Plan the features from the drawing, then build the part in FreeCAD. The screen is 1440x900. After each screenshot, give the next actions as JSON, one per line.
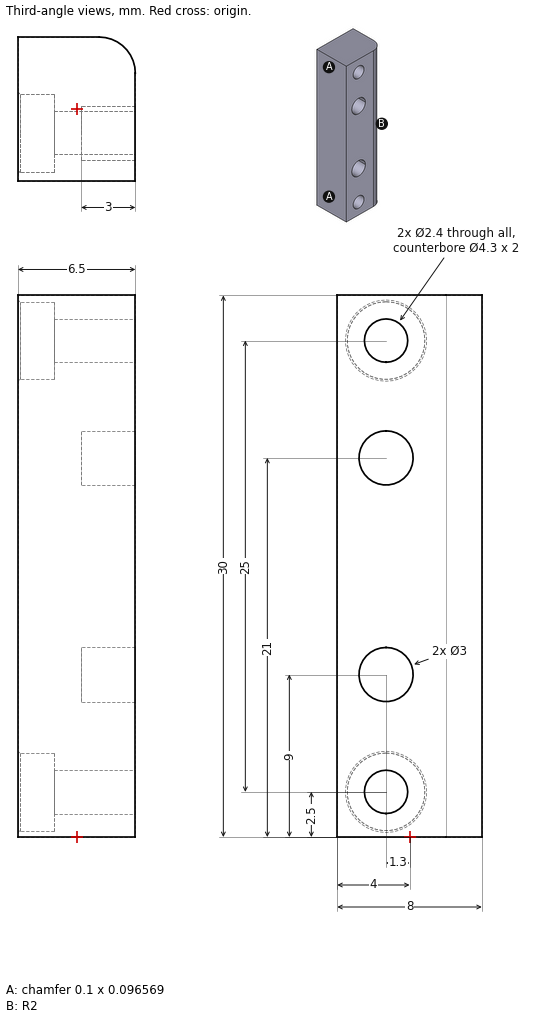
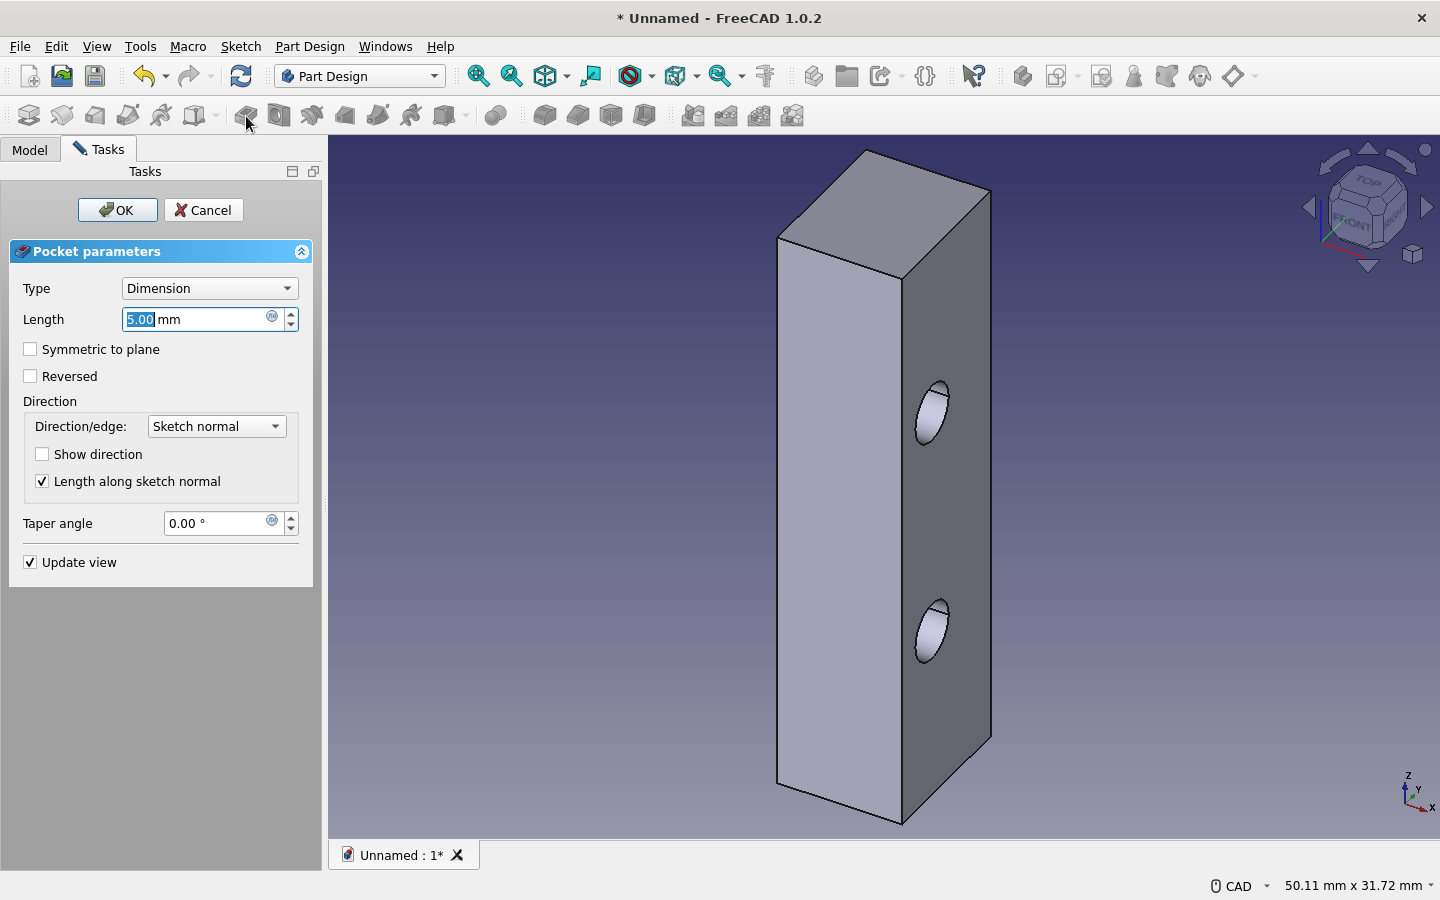
{"action": "type", "text": "3"}
{"action": "key", "text": "Tab"}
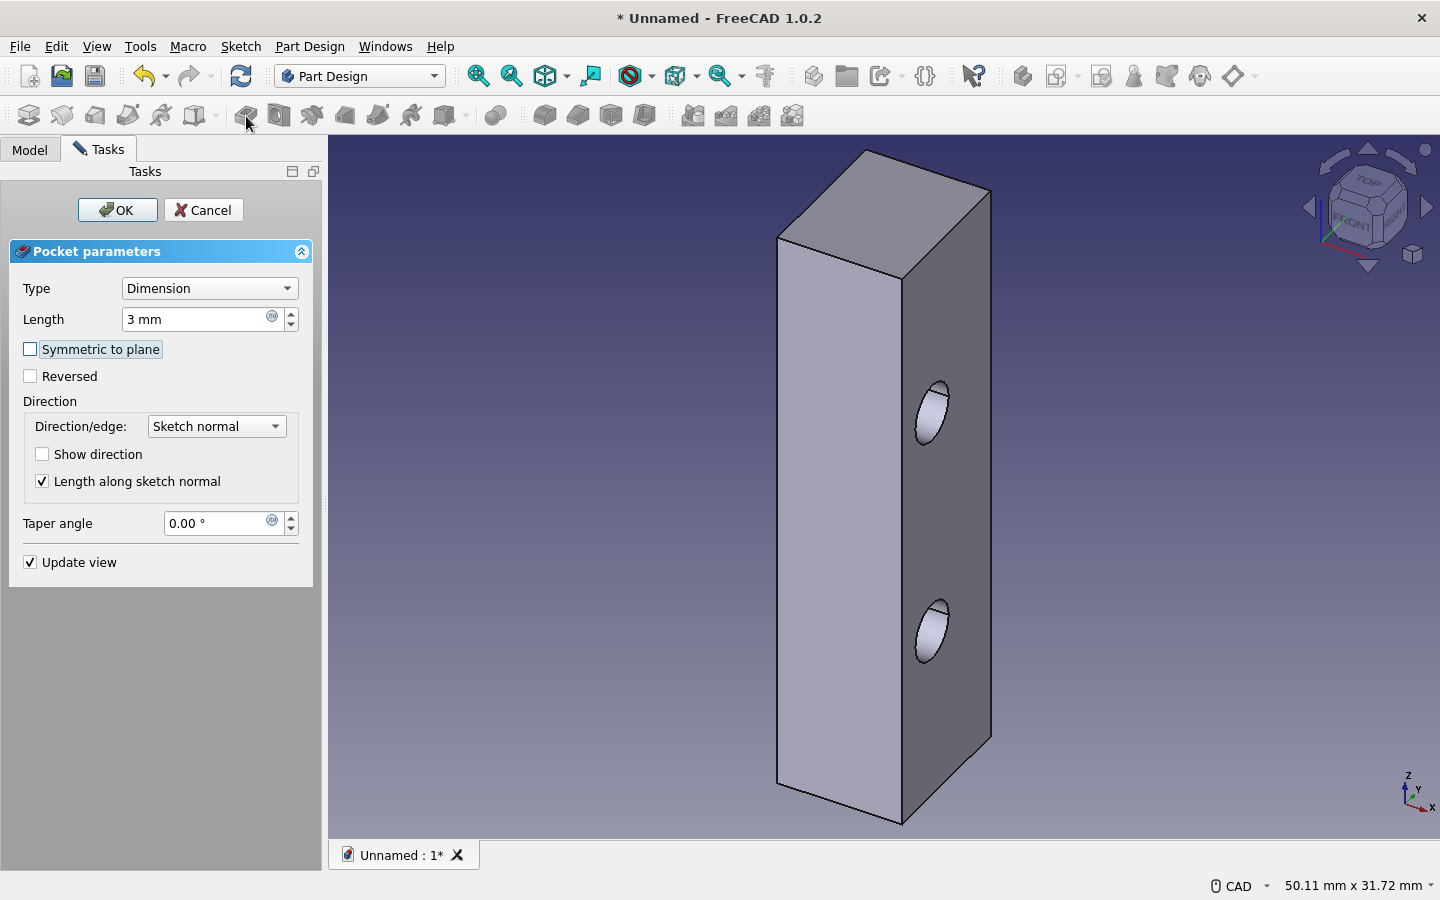
{"action": "left_click", "coordinate": [118, 210]}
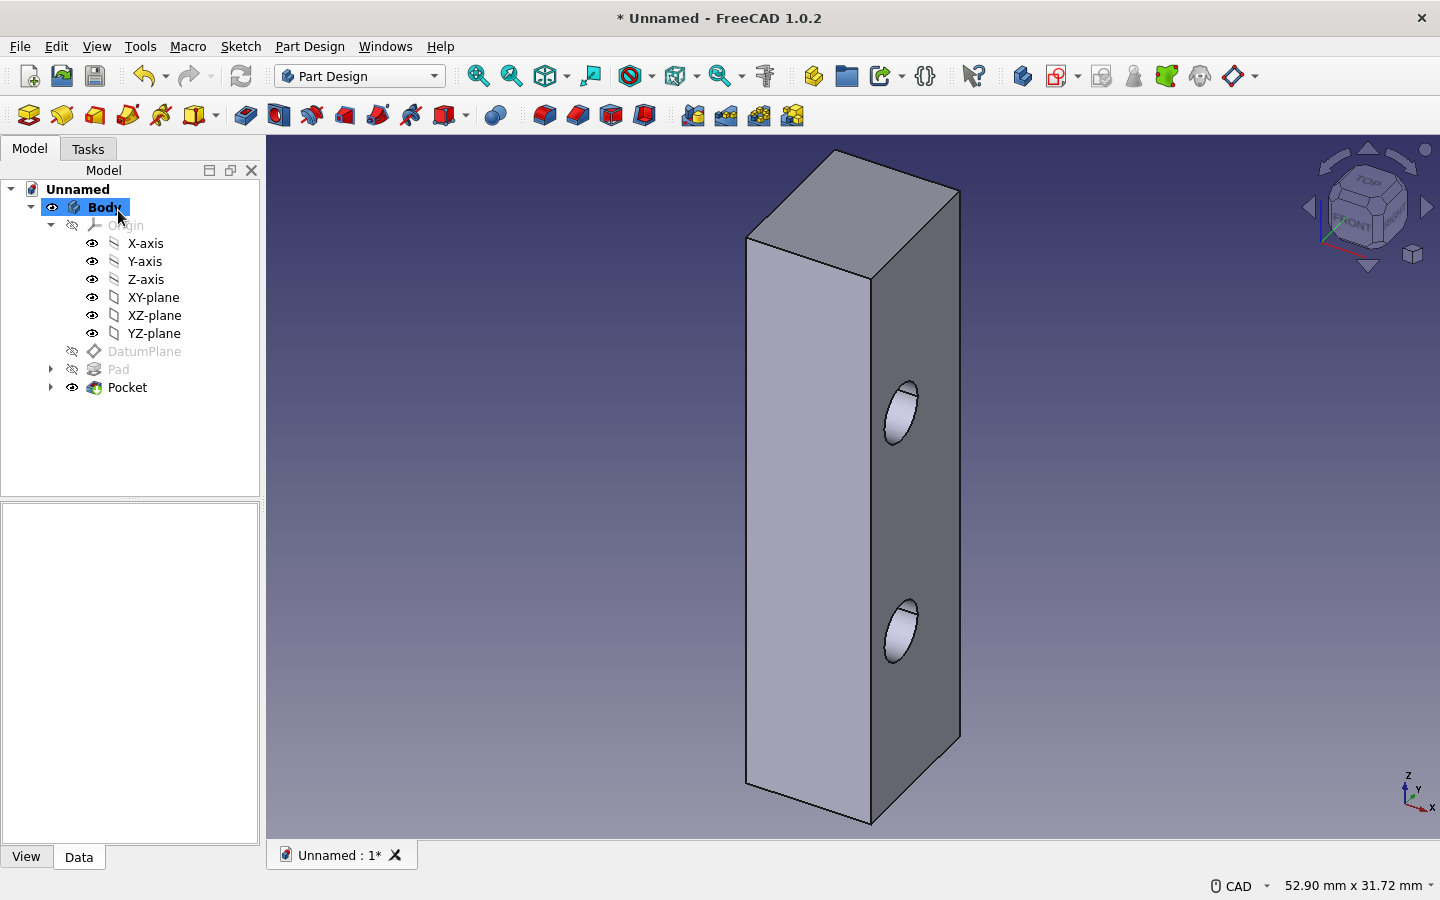
{"action": "key", "text": "6"}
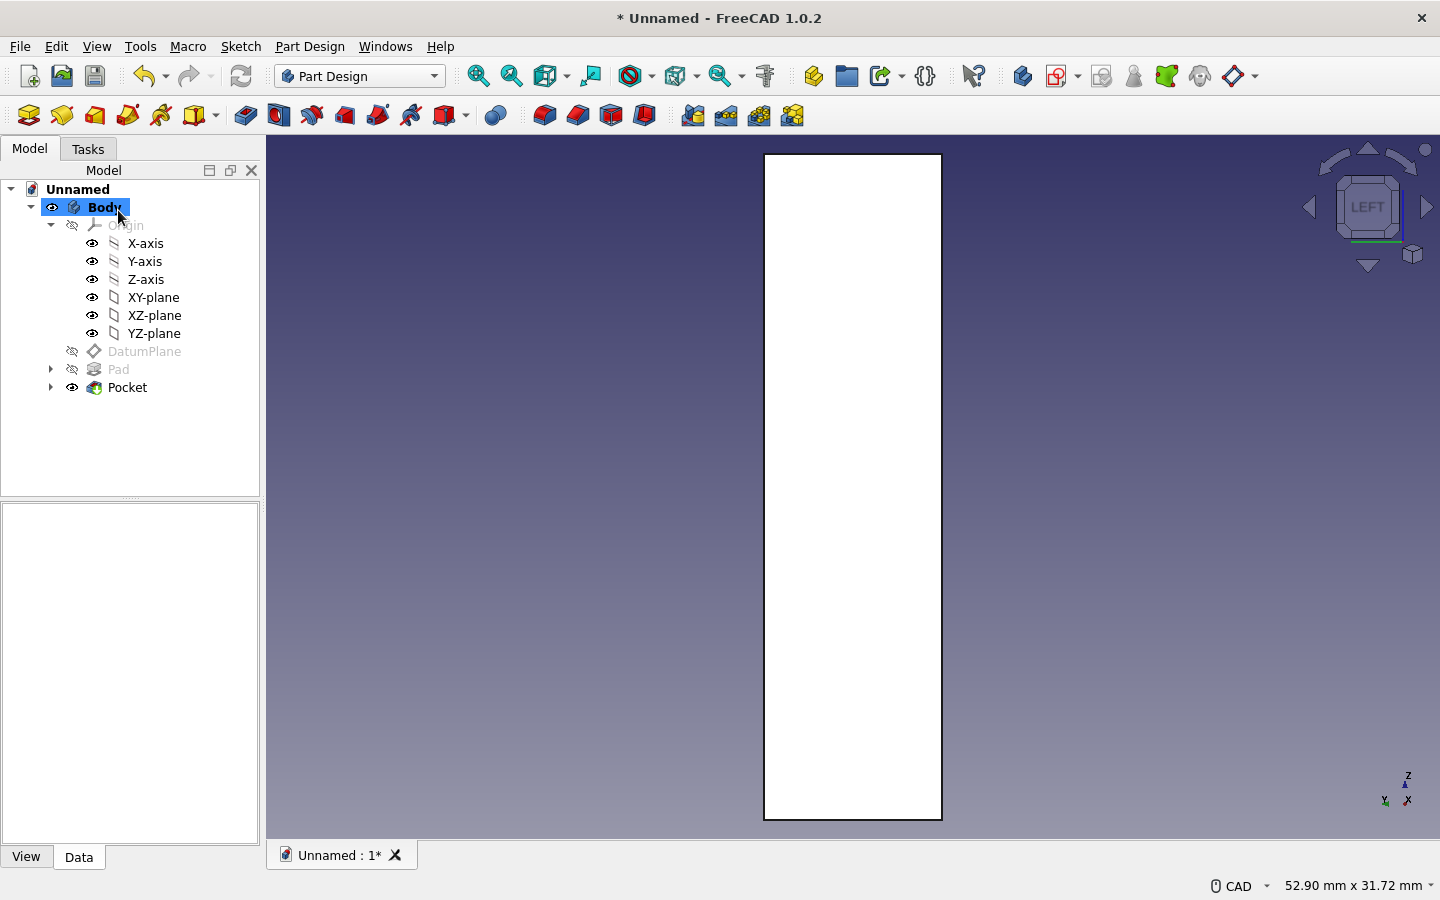
{"action": "left_click", "coordinate": [853, 296]}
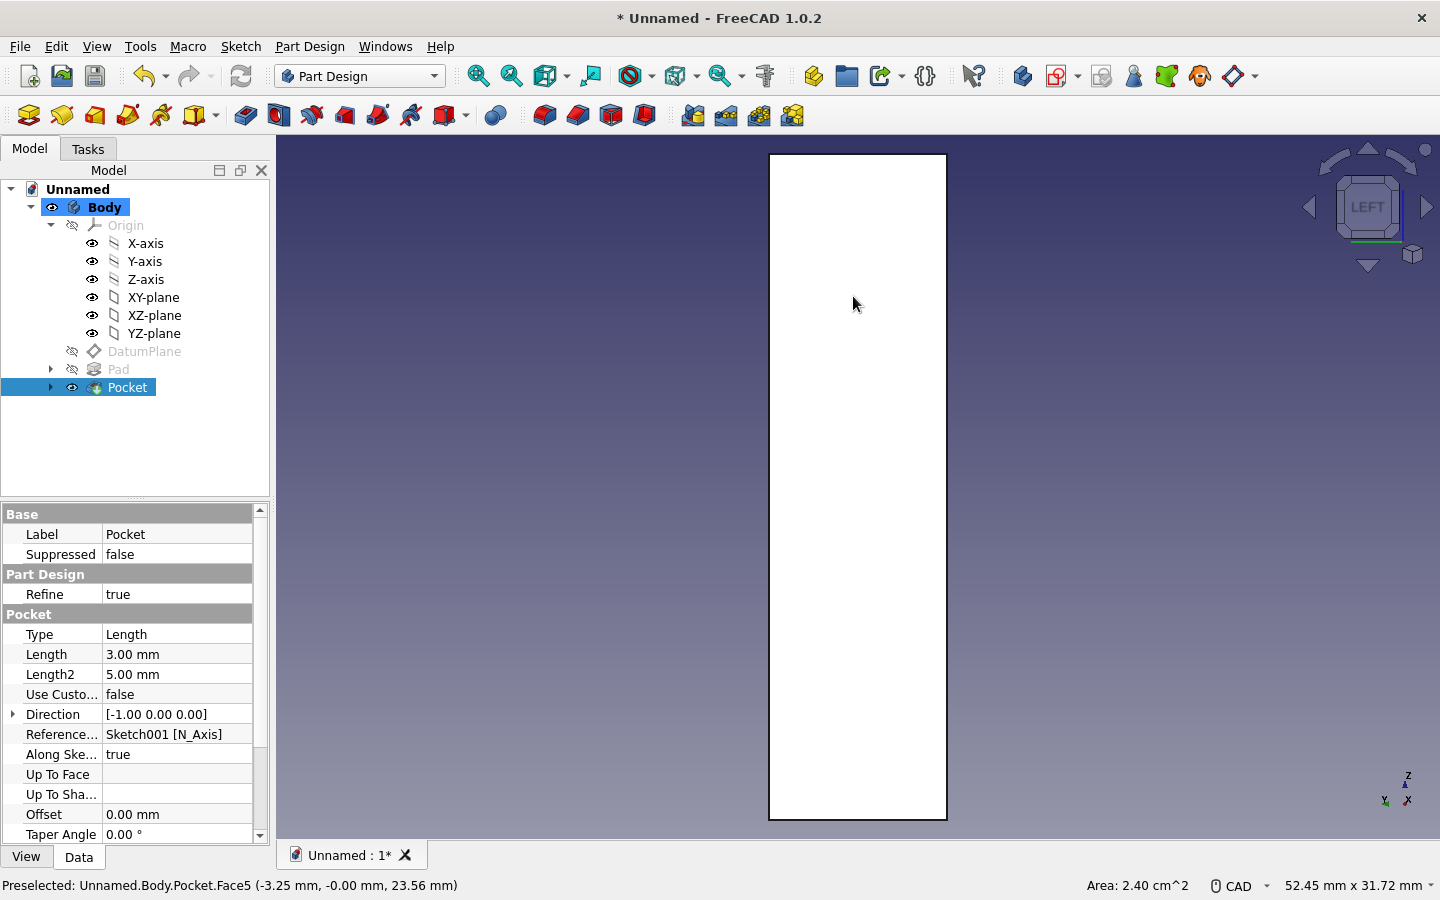
{"action": "left_click", "coordinate": [1056, 76]}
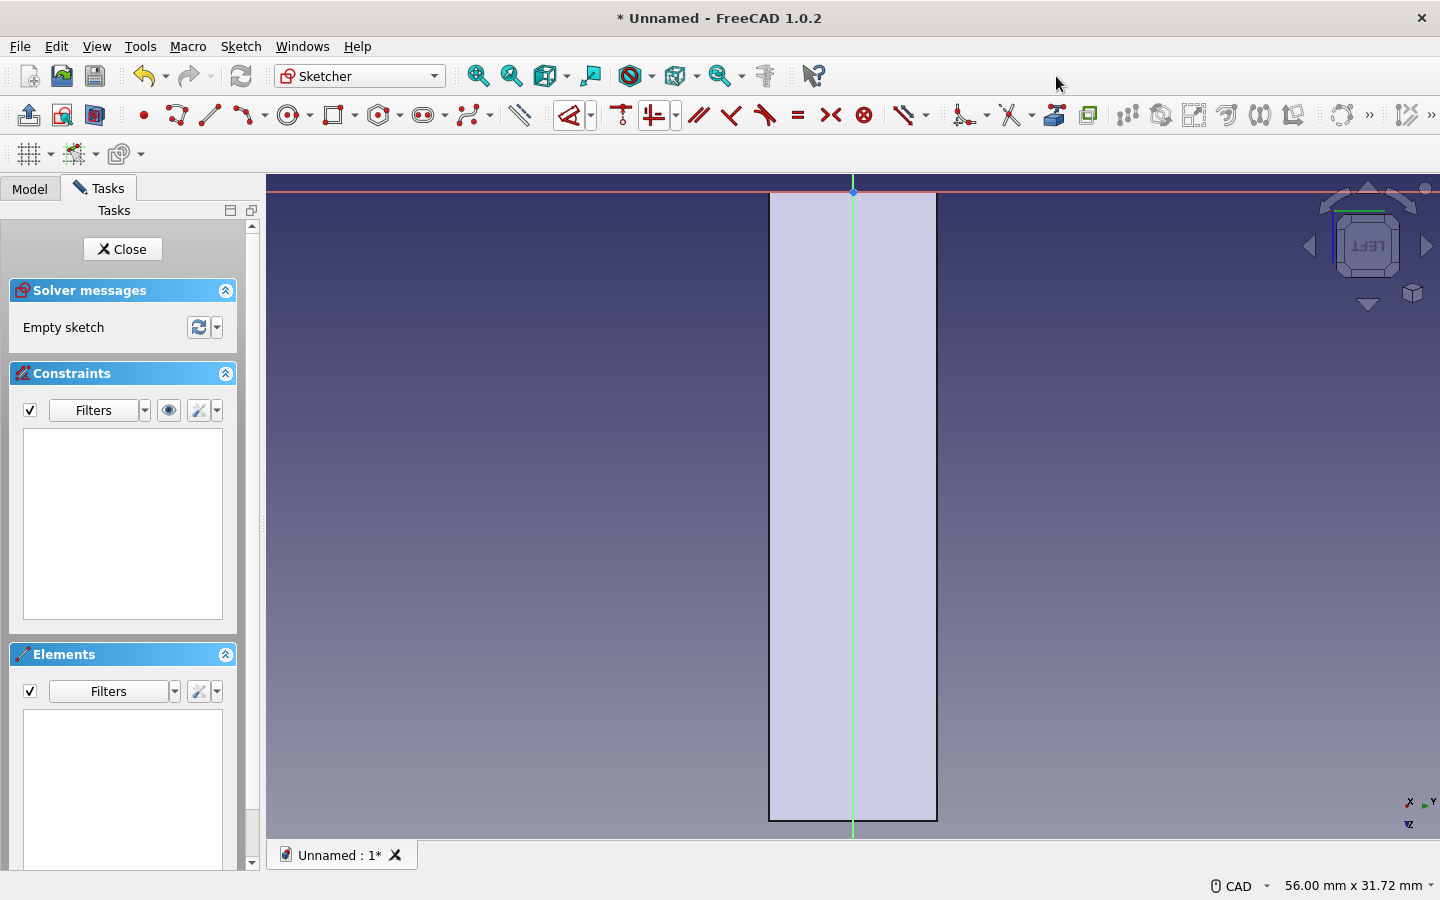
{"action": "scroll", "coordinate": [699, 534], "scroll_direction": "down", "scroll_amount": 2}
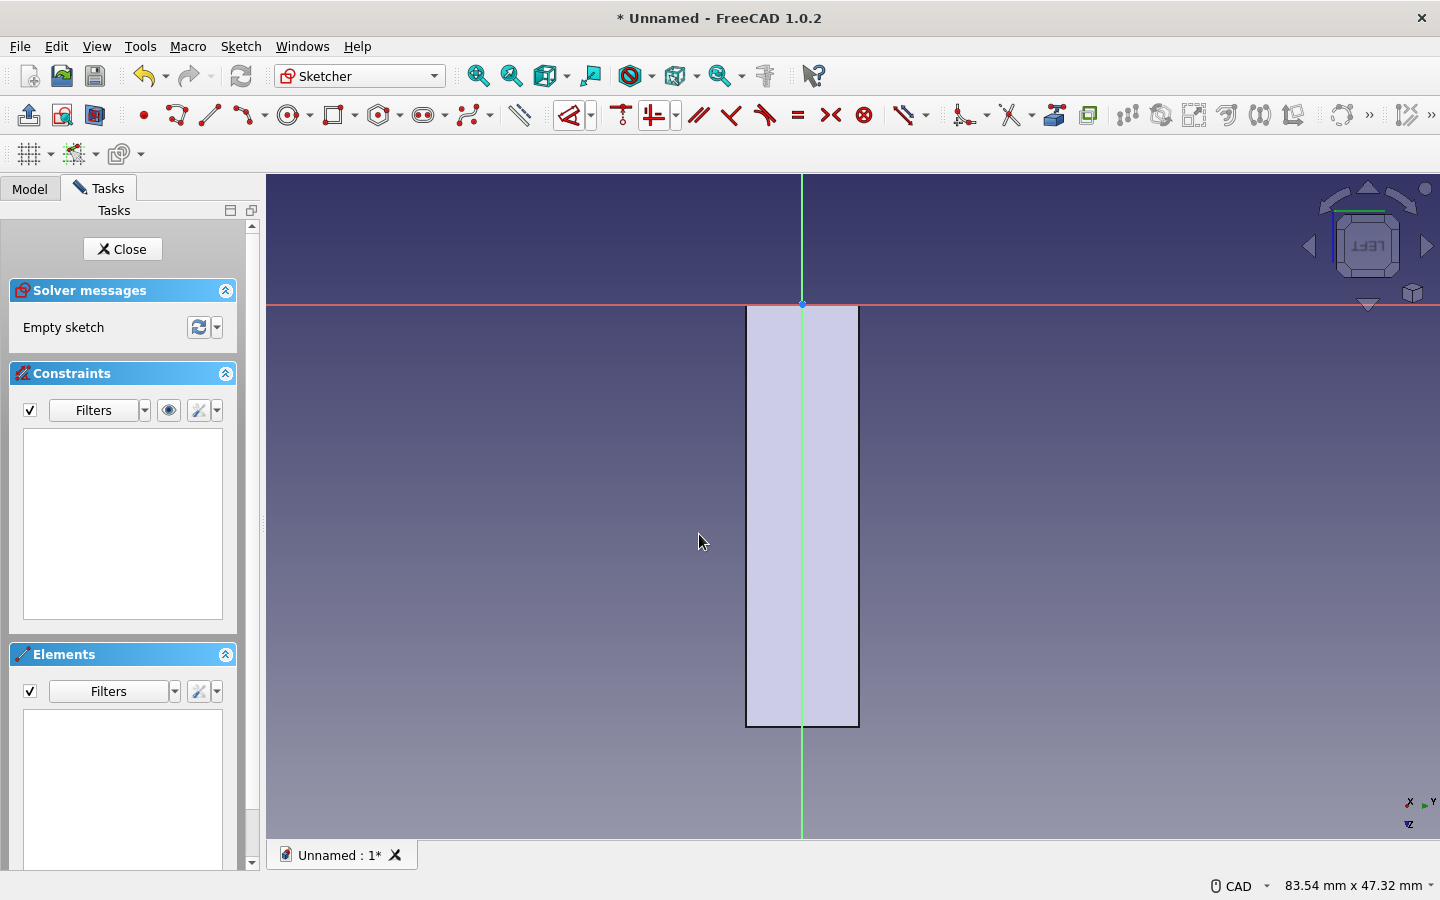
{"action": "left_click", "coordinate": [288, 116]}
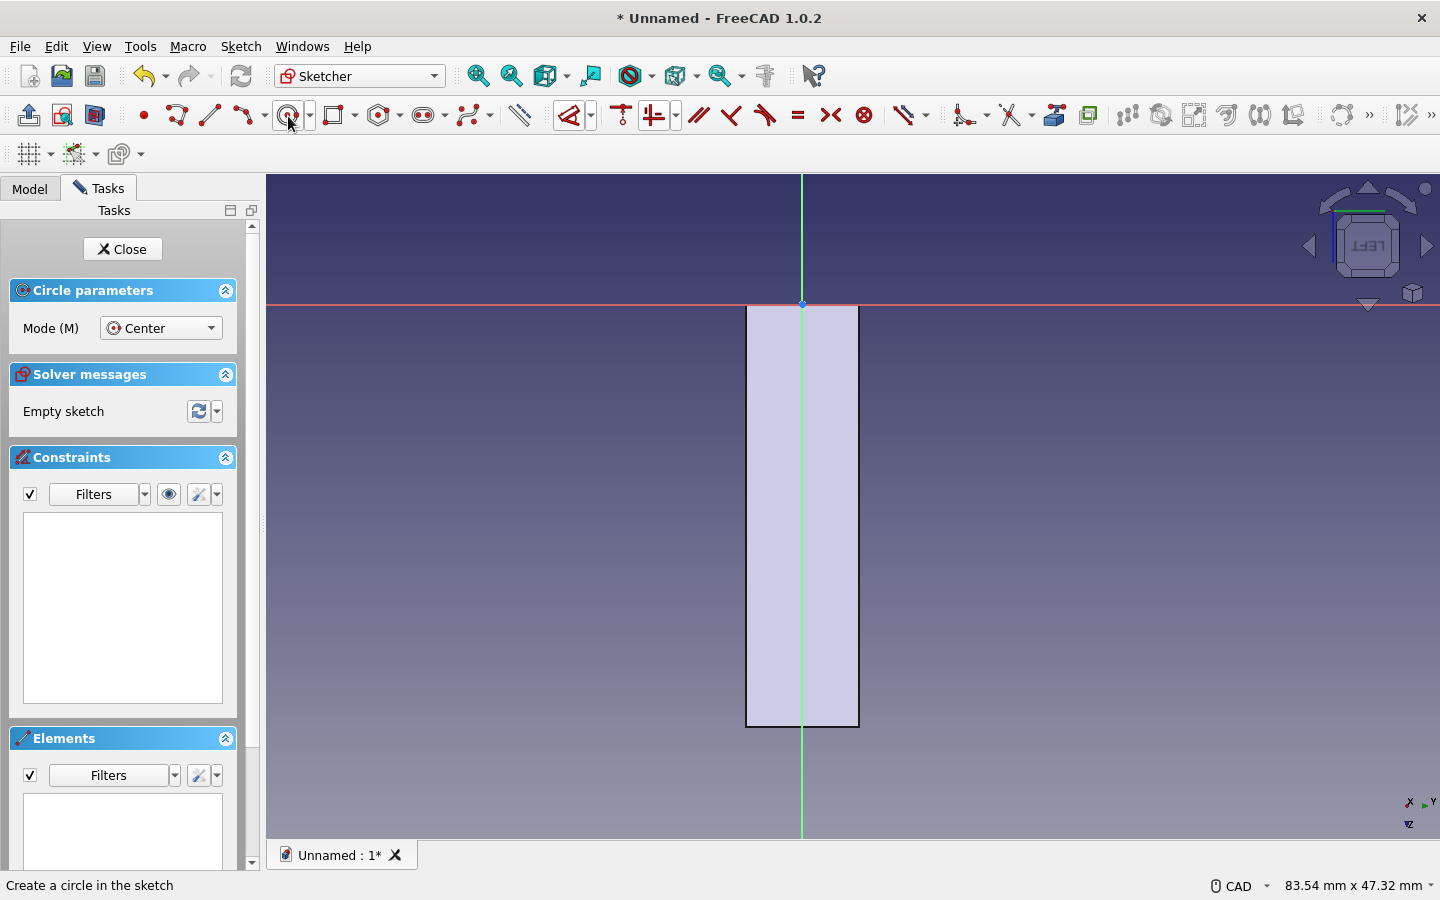
{"action": "scroll", "coordinate": [784, 691], "scroll_direction": "up", "scroll_amount": 2}